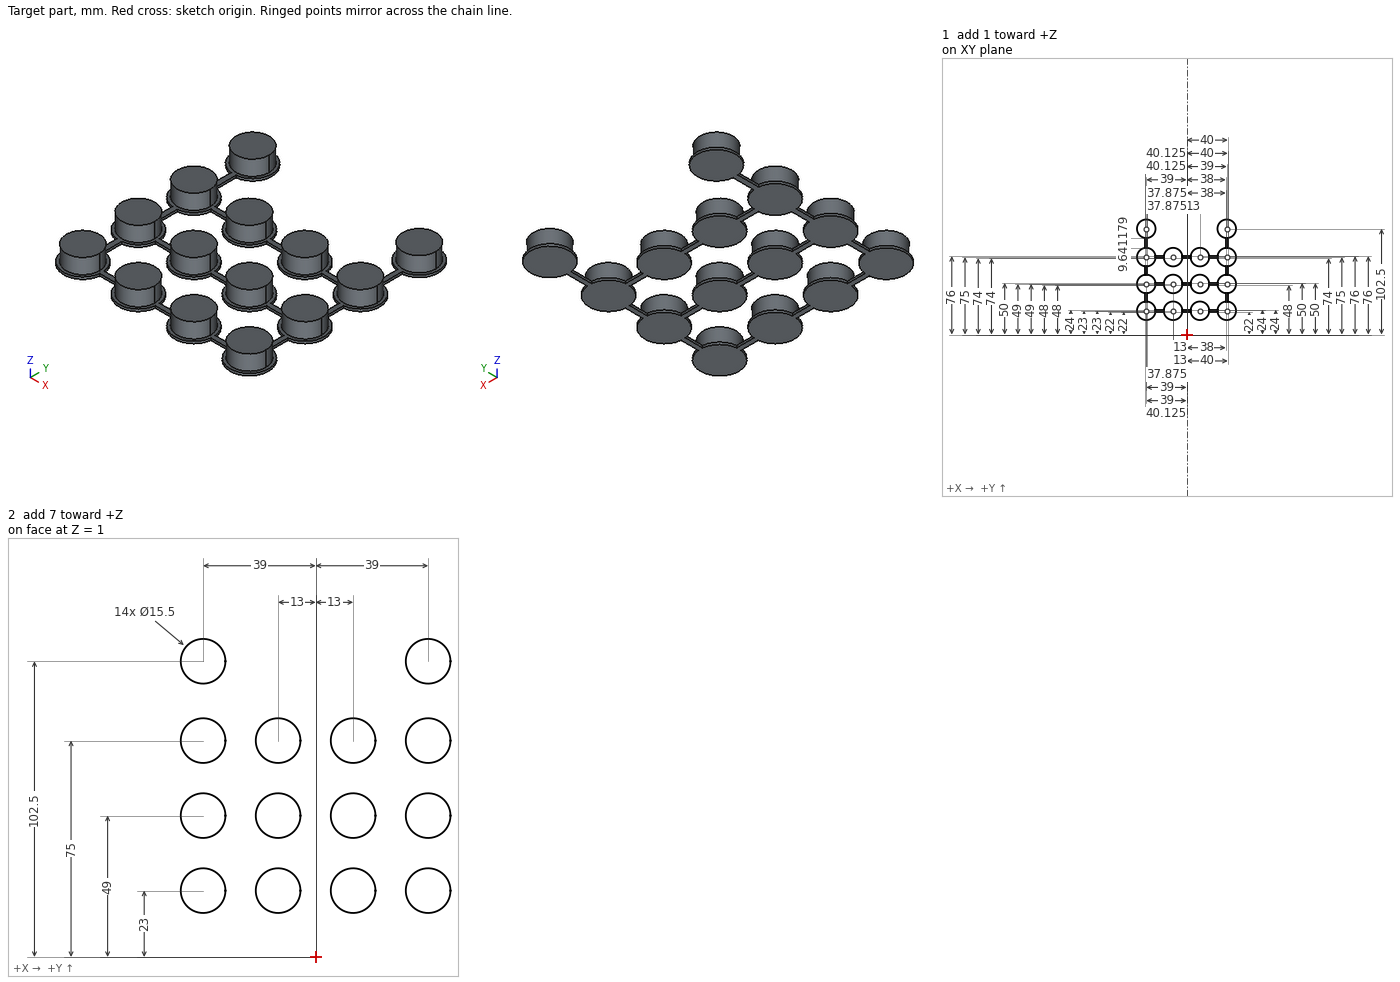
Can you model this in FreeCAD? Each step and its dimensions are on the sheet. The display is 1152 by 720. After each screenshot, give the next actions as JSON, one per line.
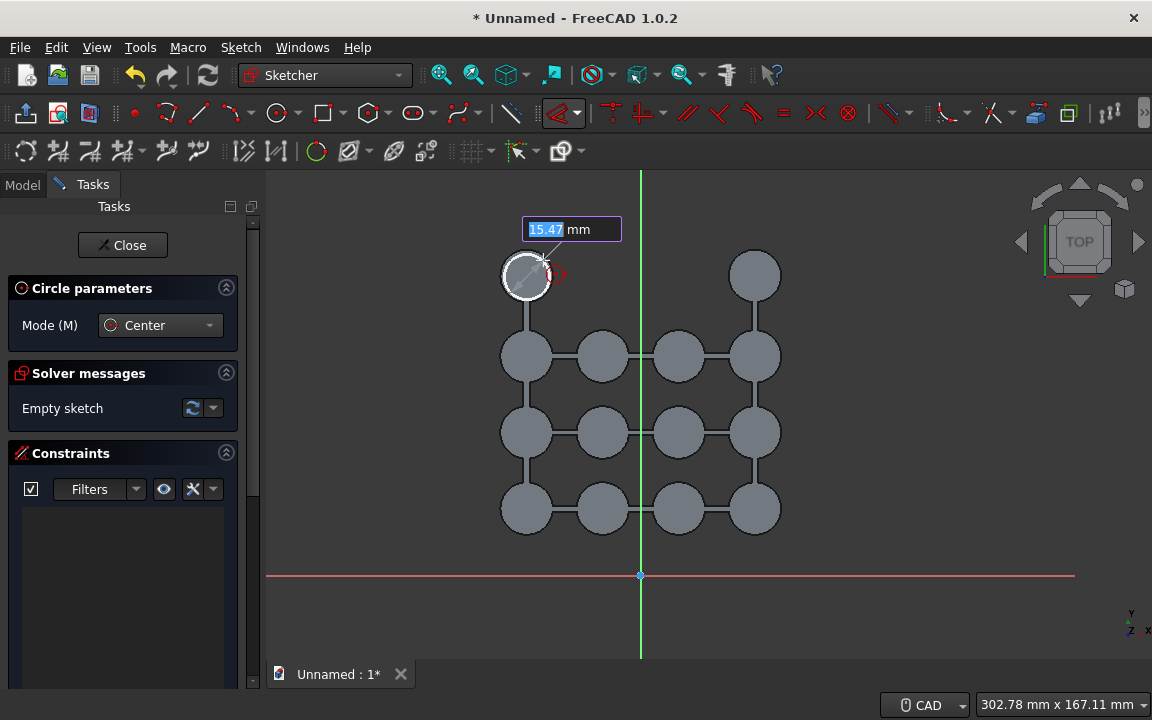
{"action": "type", "text": "15.5"}
{"action": "key", "text": "Return"}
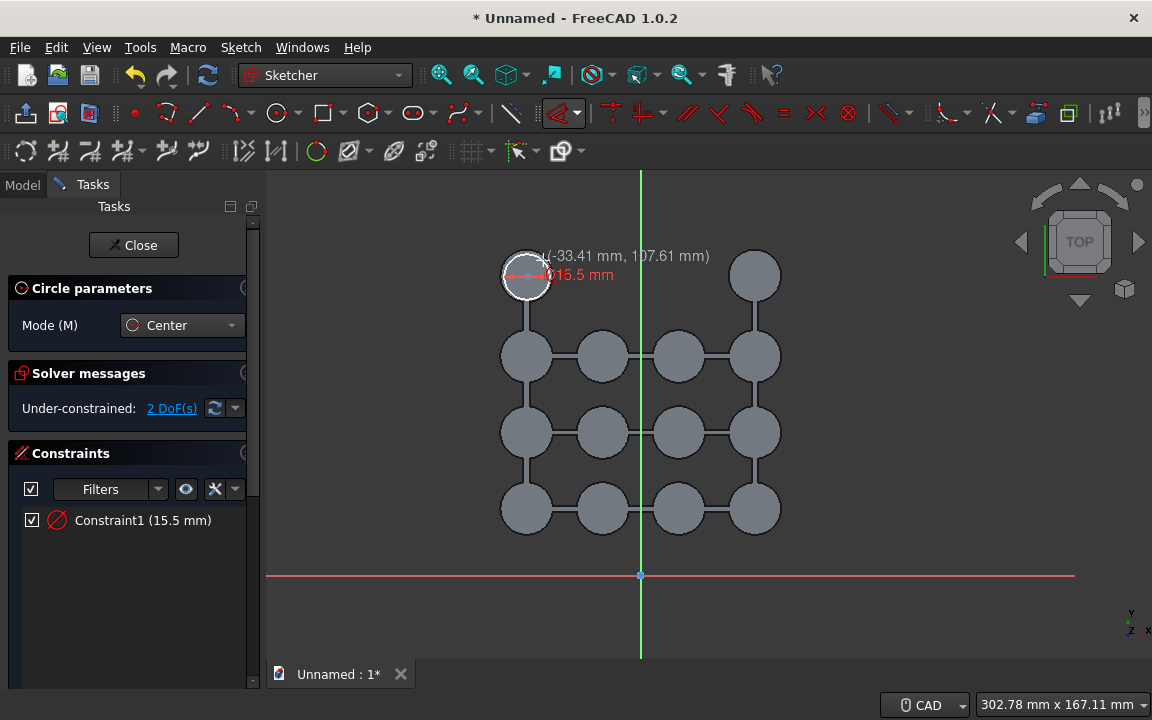
{"action": "left_click", "coordinate": [527, 356]}
{"action": "mouse_move", "coordinate": [543, 340]}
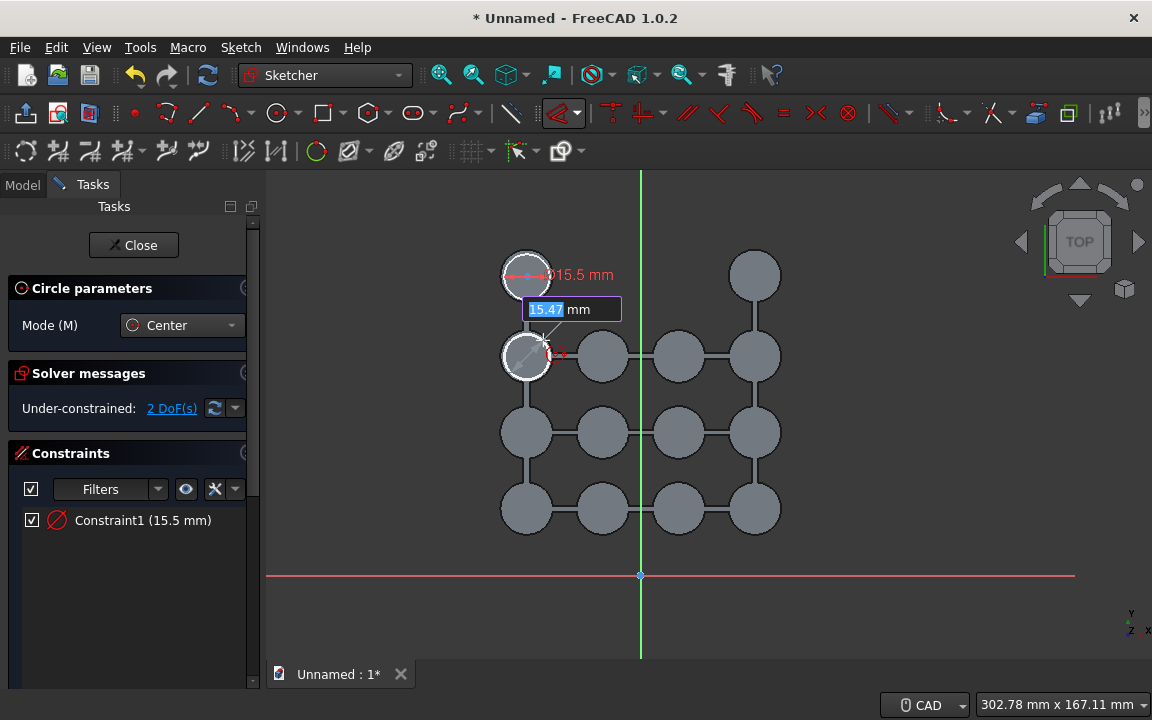
{"action": "type", "text": "15.5"}
{"action": "key", "text": "Return"}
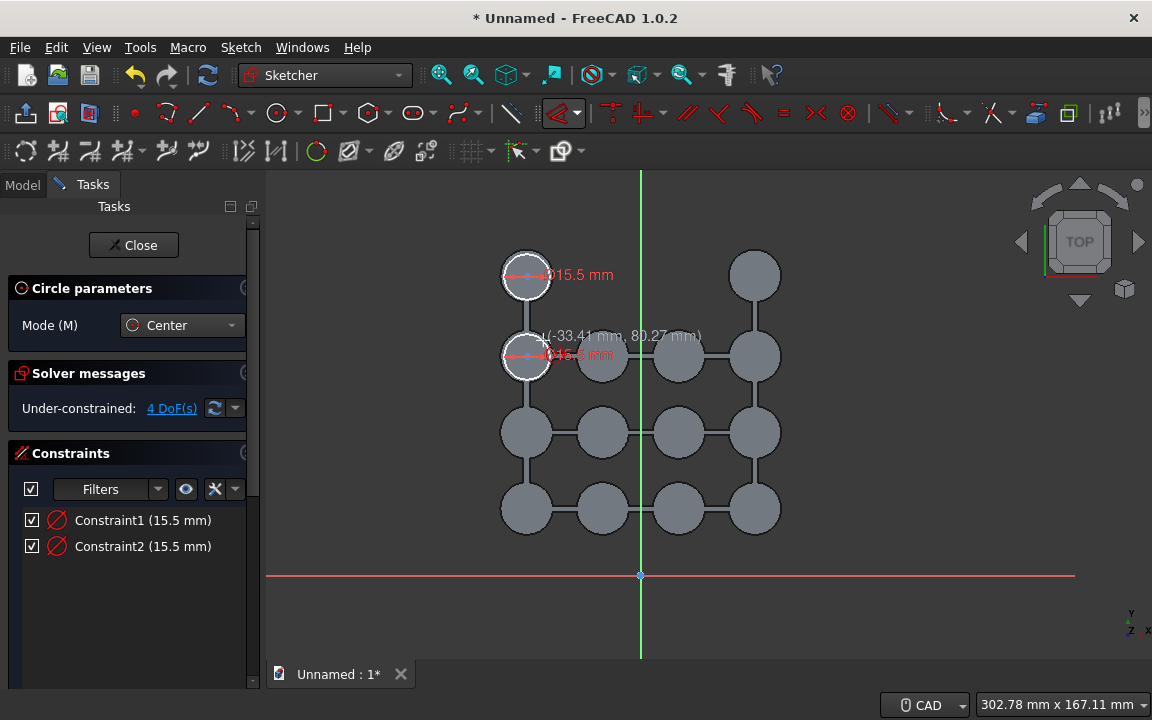
{"action": "left_click", "coordinate": [527, 432]}
{"action": "mouse_move", "coordinate": [543, 416]}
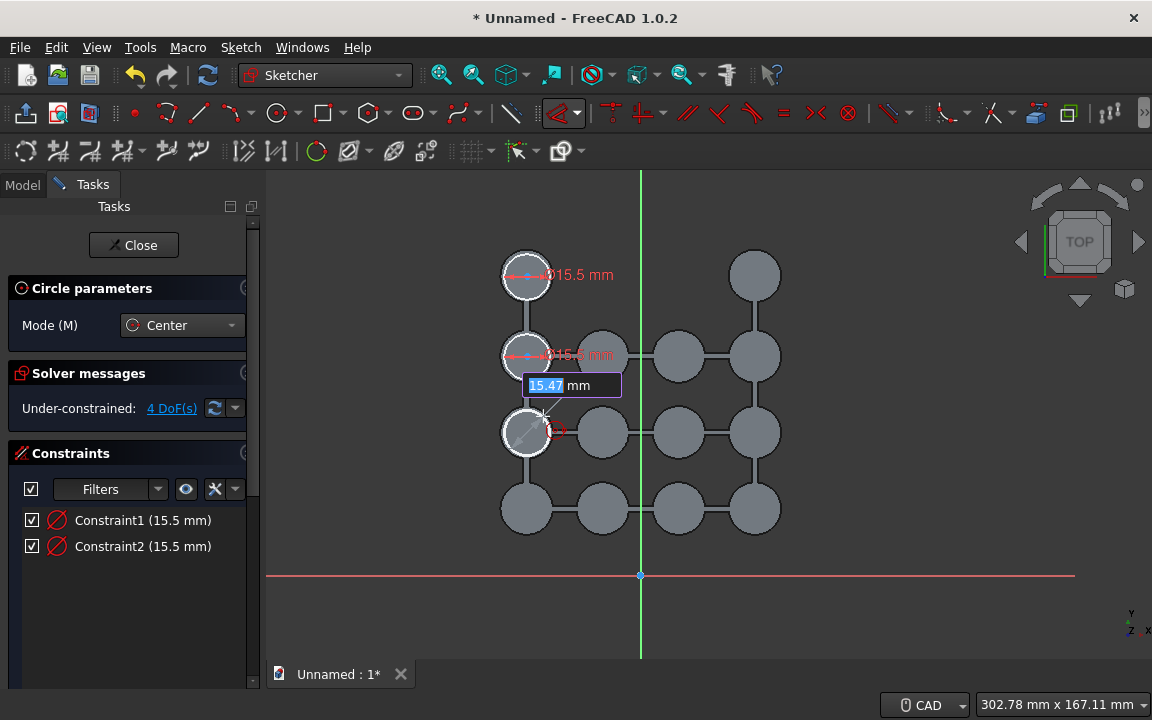
{"action": "type", "text": "15.5"}
{"action": "key", "text": "Return"}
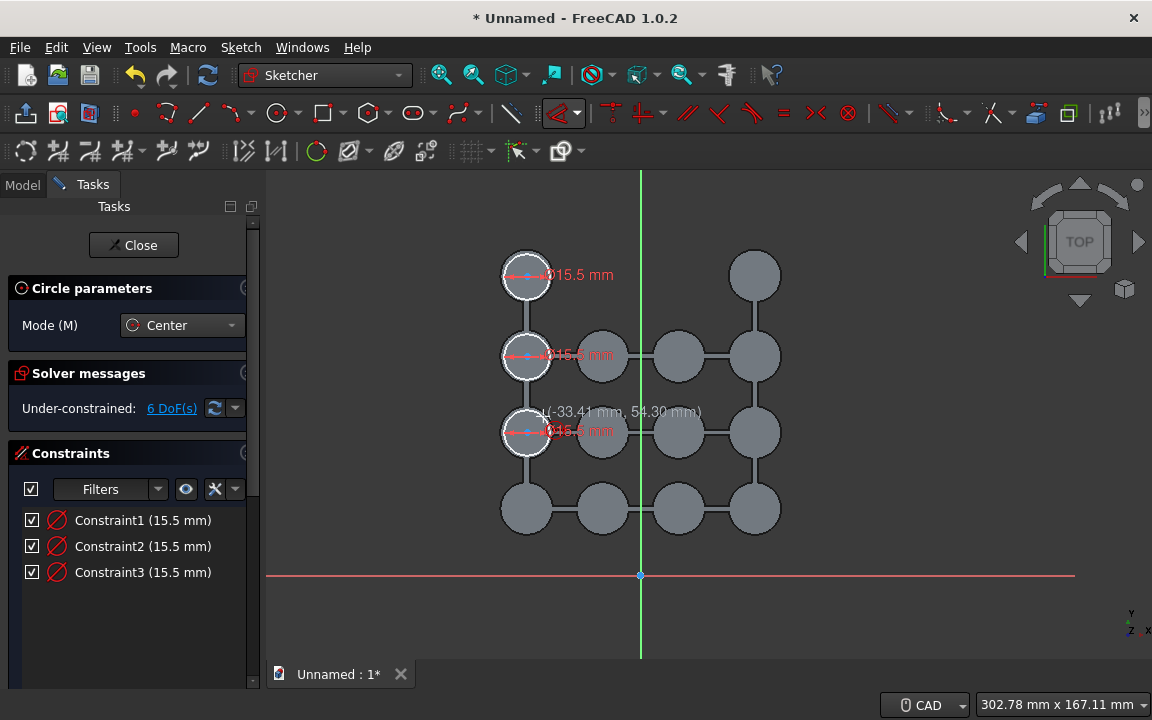
{"action": "left_click", "coordinate": [527, 509]}
{"action": "mouse_move", "coordinate": [543, 493]}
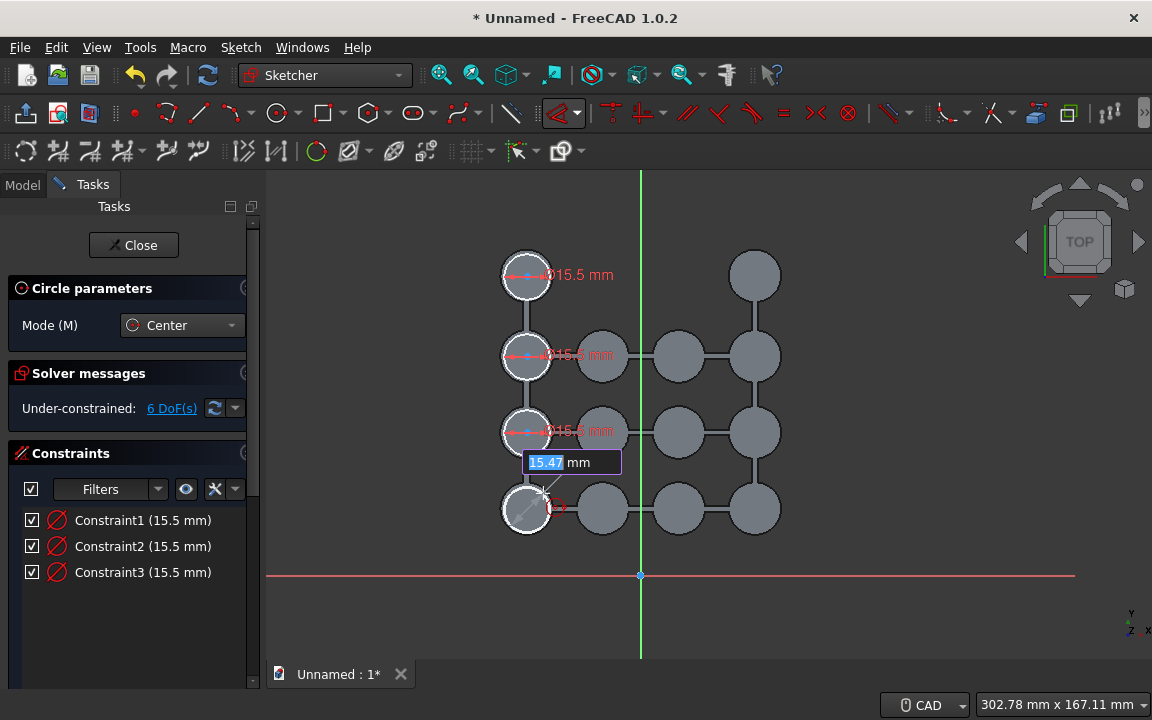
{"action": "type", "text": "15.5"}
{"action": "key", "text": "Return"}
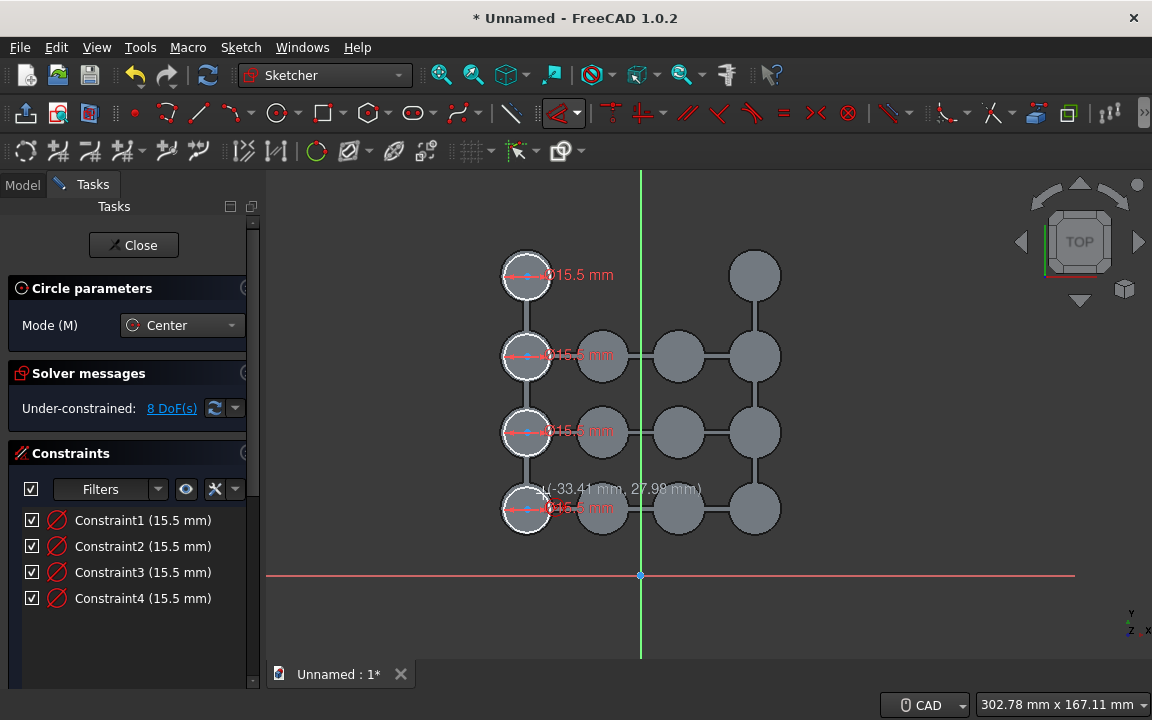
{"action": "left_click", "coordinate": [603, 356]}
{"action": "mouse_move", "coordinate": [619, 340]}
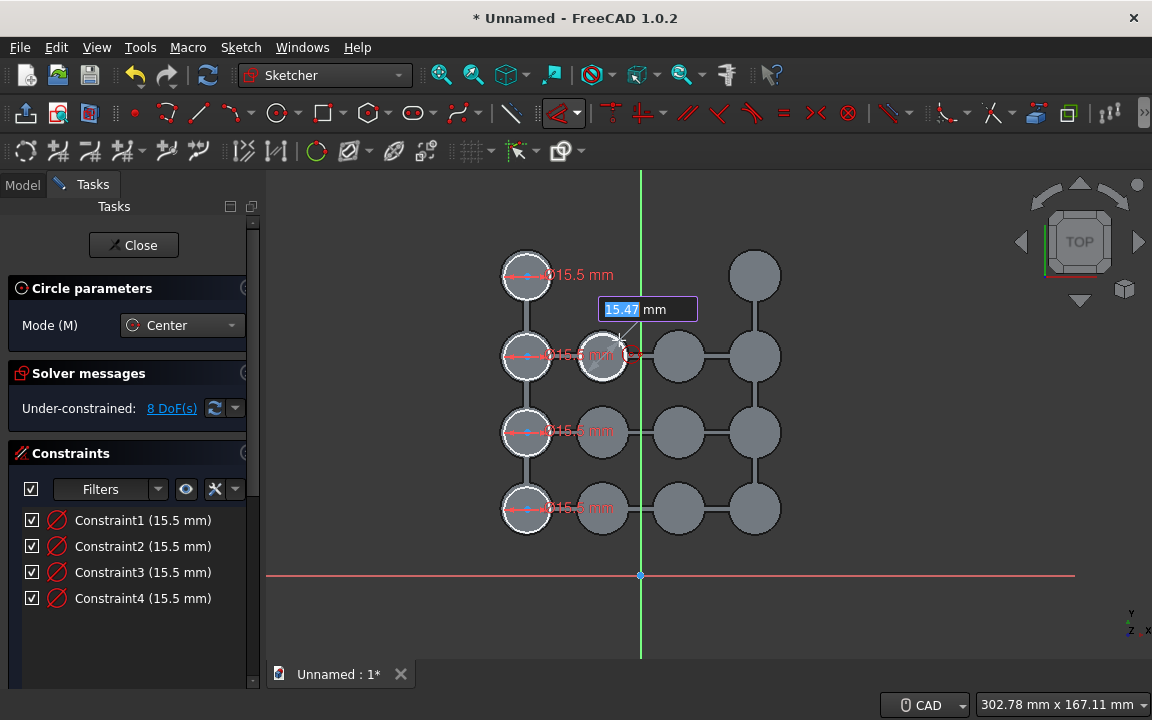
{"action": "type", "text": "15.5"}
{"action": "key", "text": "Return"}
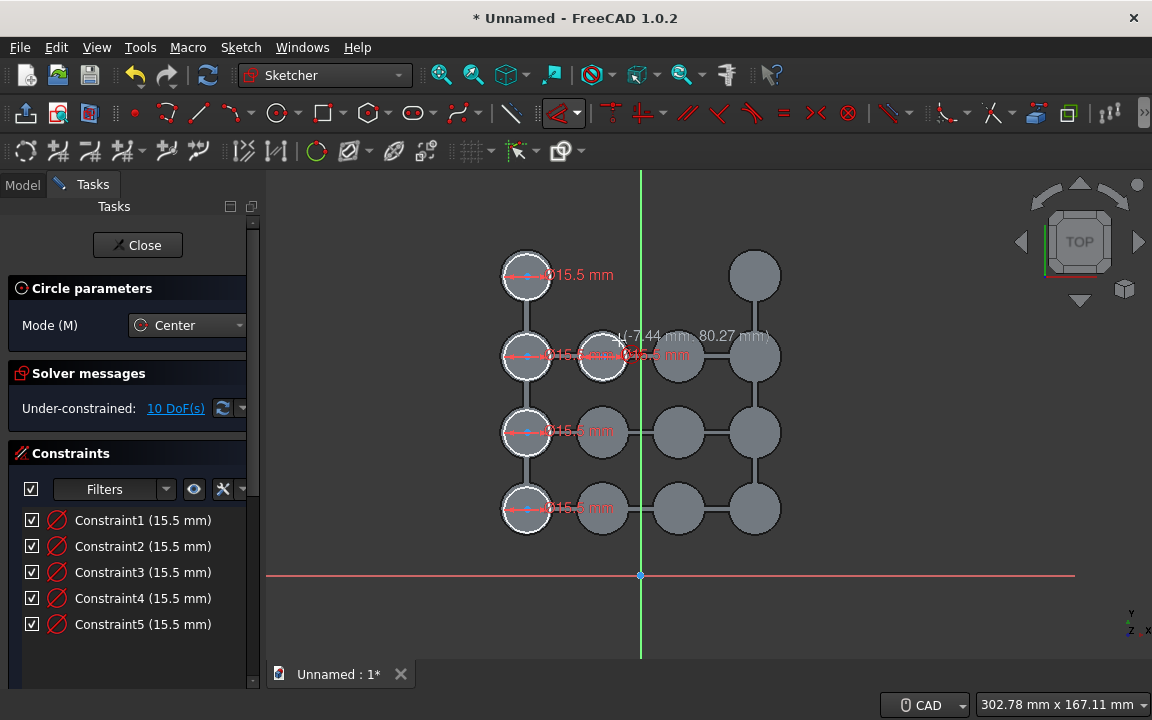
{"action": "left_click", "coordinate": [603, 432]}
{"action": "mouse_move", "coordinate": [619, 416]}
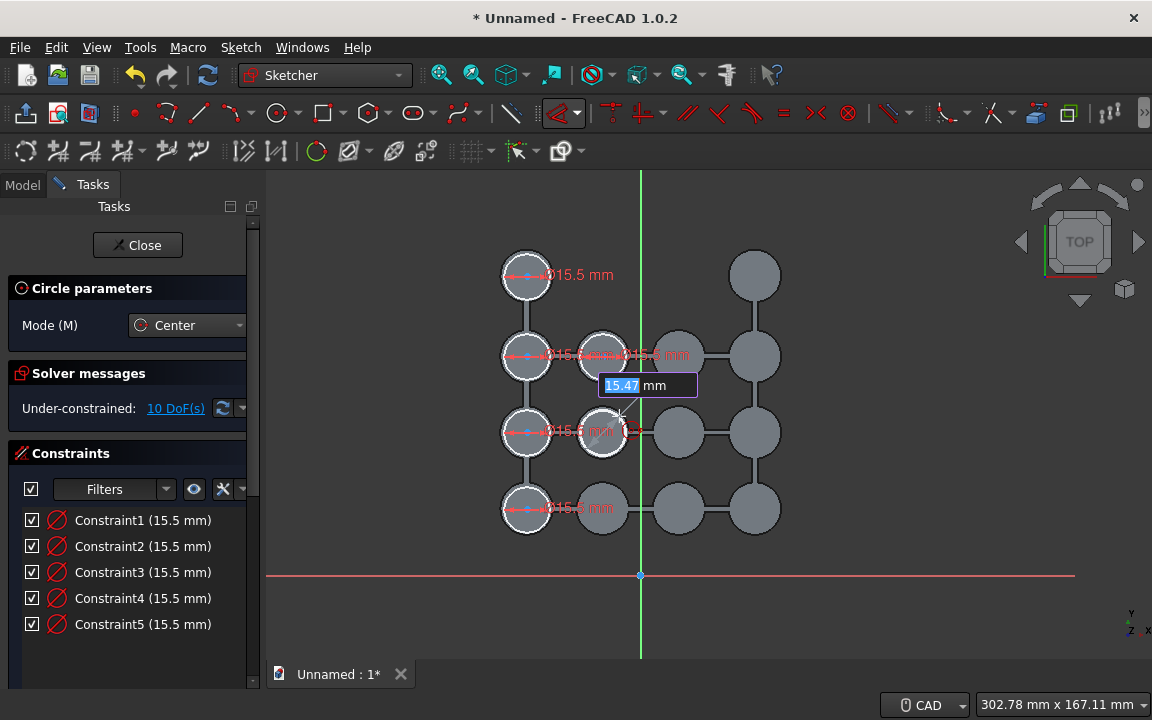
{"action": "type", "text": "15.5"}
{"action": "key", "text": "Return"}